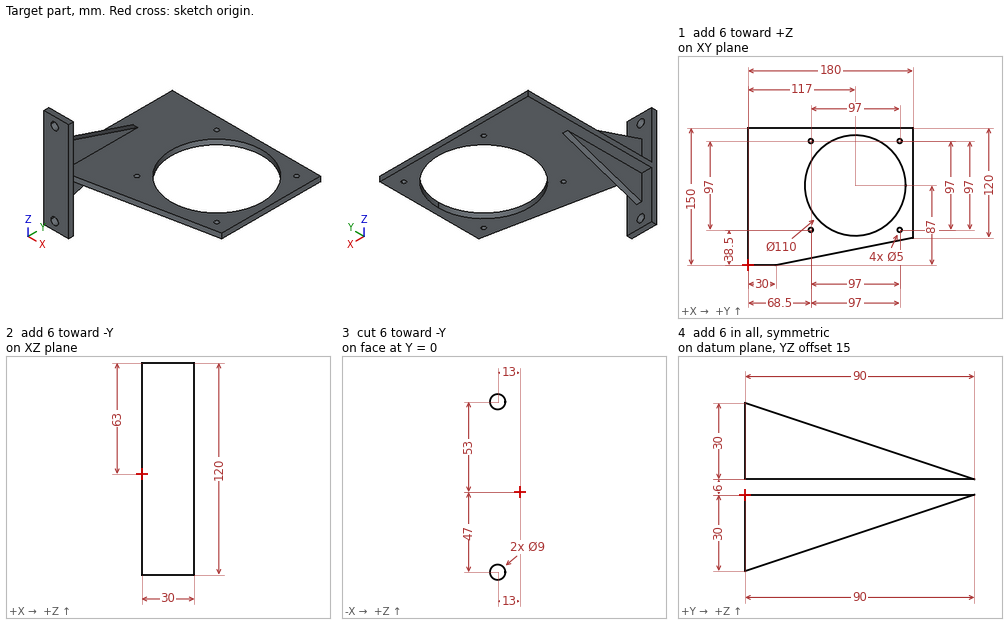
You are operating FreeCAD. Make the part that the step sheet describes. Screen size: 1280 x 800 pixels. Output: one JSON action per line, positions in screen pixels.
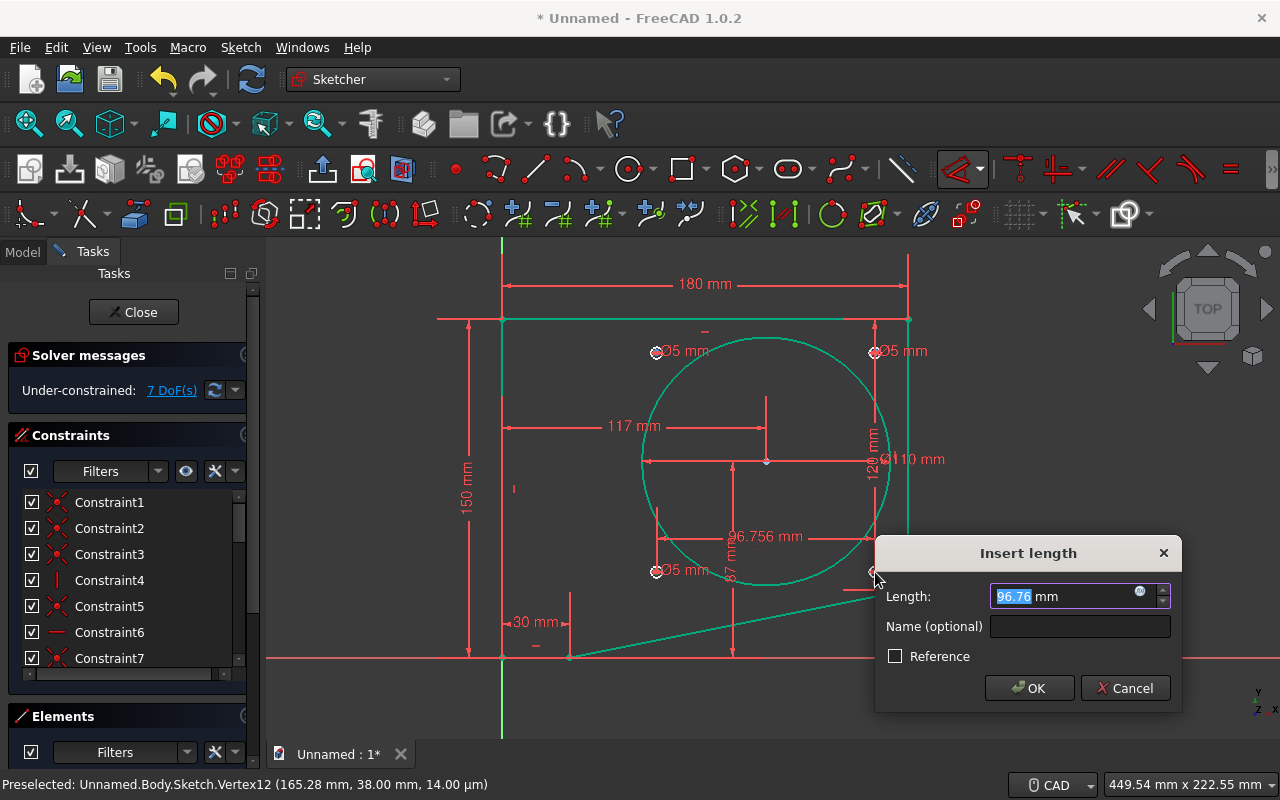
{"action": "type", "text": "97"}
{"action": "key", "text": "Return"}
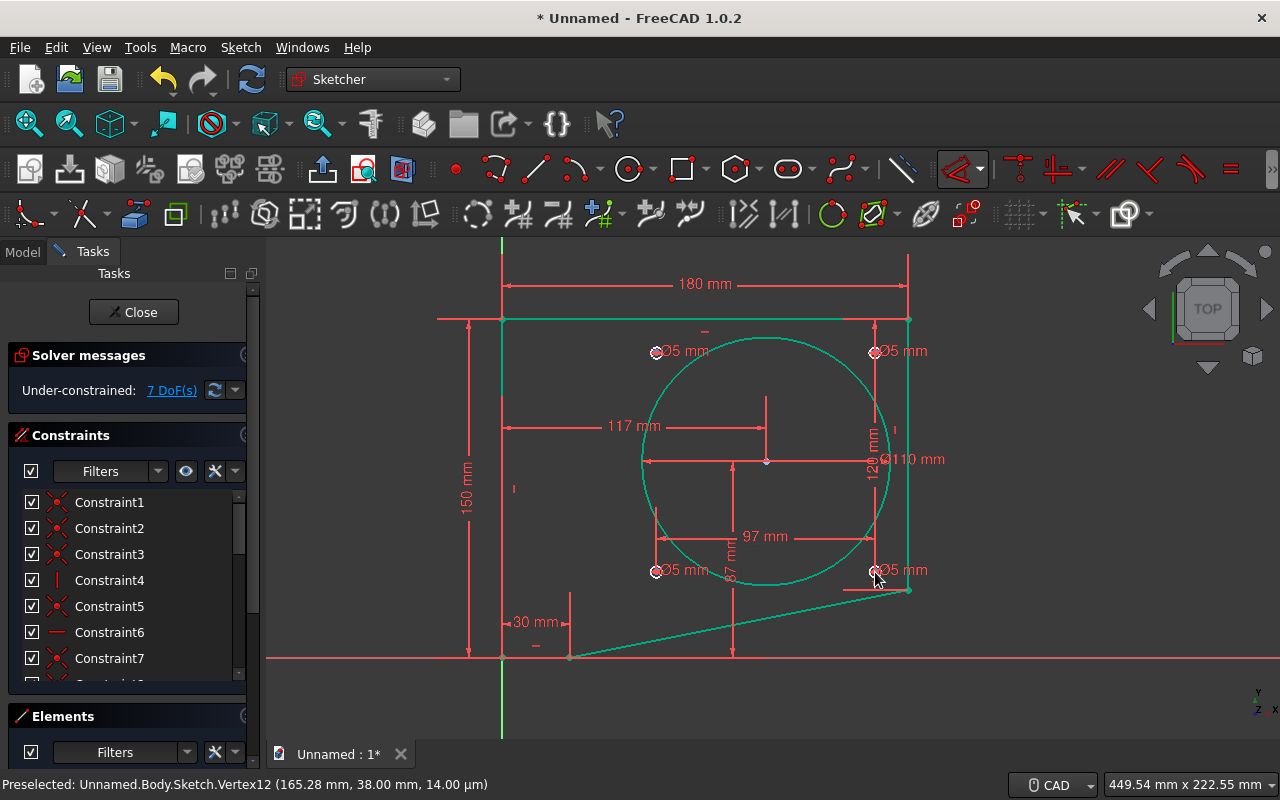
{"action": "left_click", "coordinate": [875, 572]}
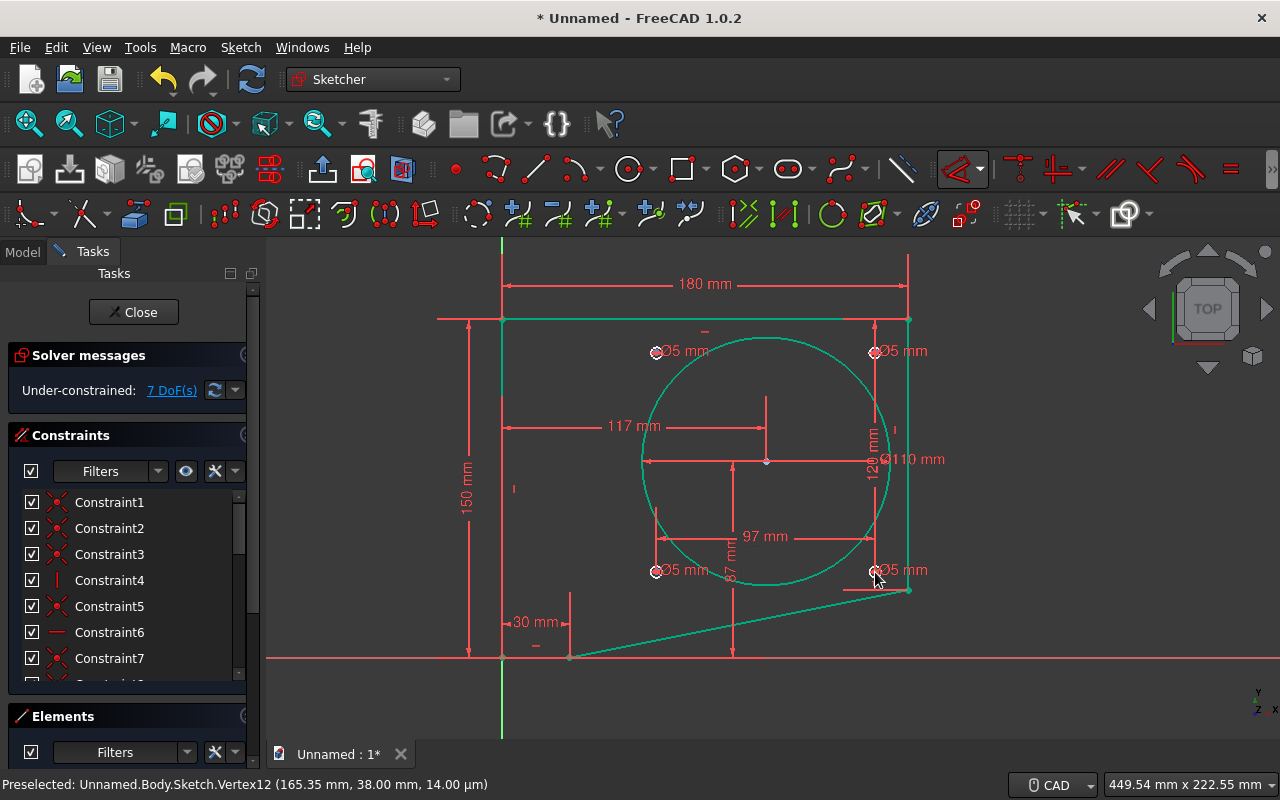
{"action": "left_click", "coordinate": [657, 353]}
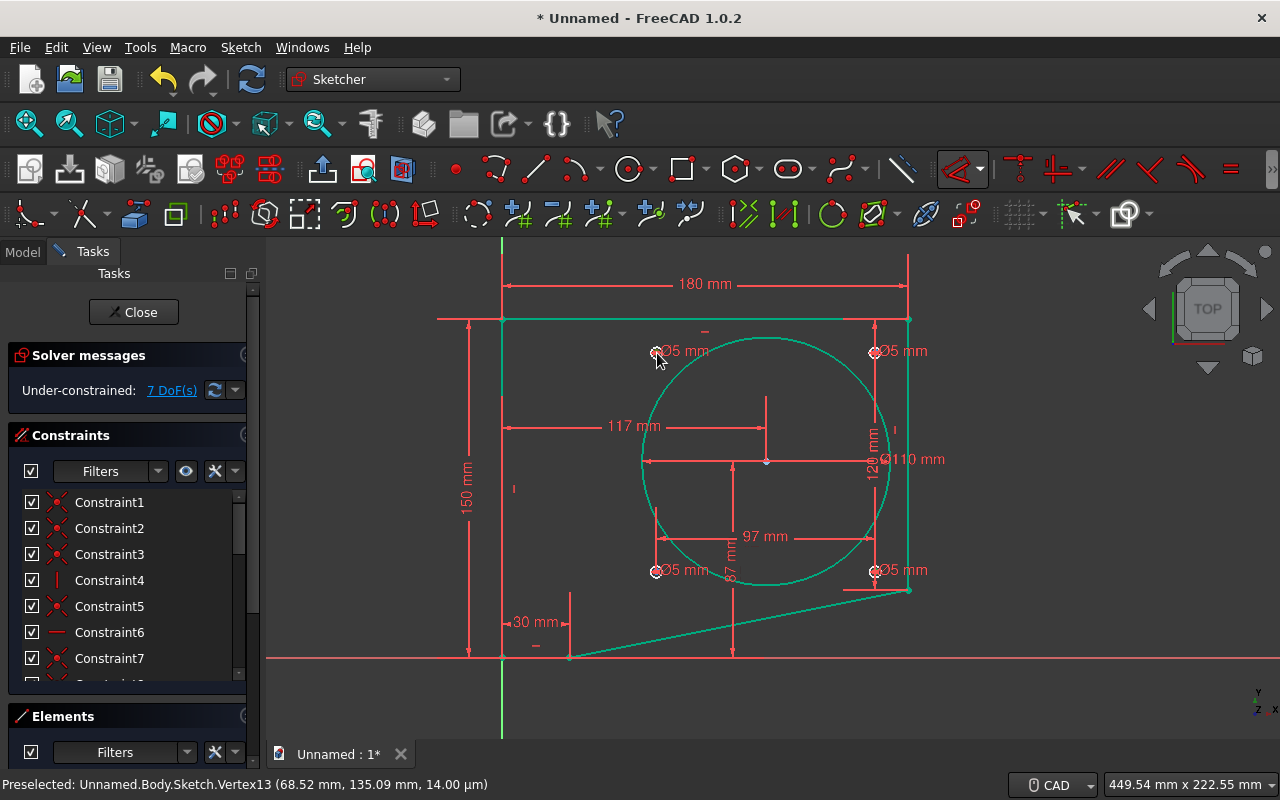
{"action": "key", "text": "l"}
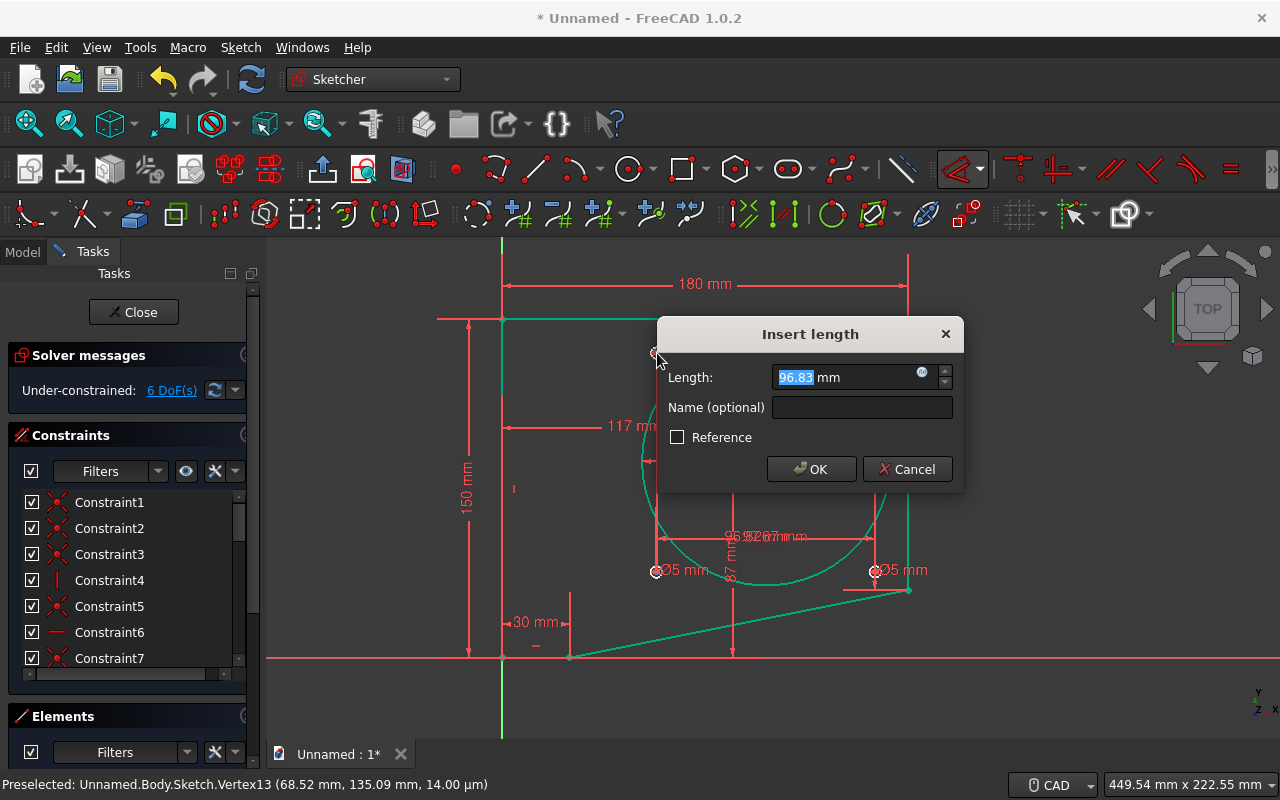
{"action": "type", "text": "97"}
{"action": "key", "text": "Return"}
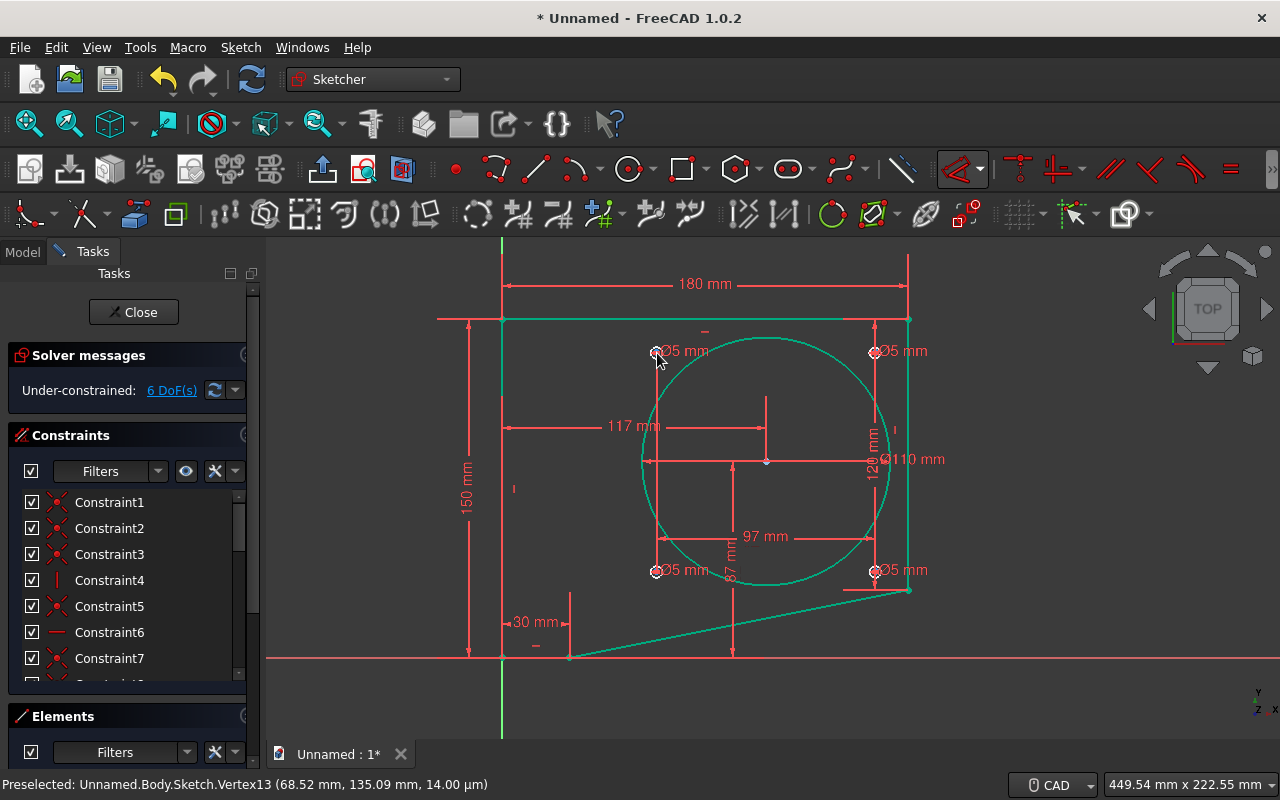
{"action": "left_click", "coordinate": [657, 572]}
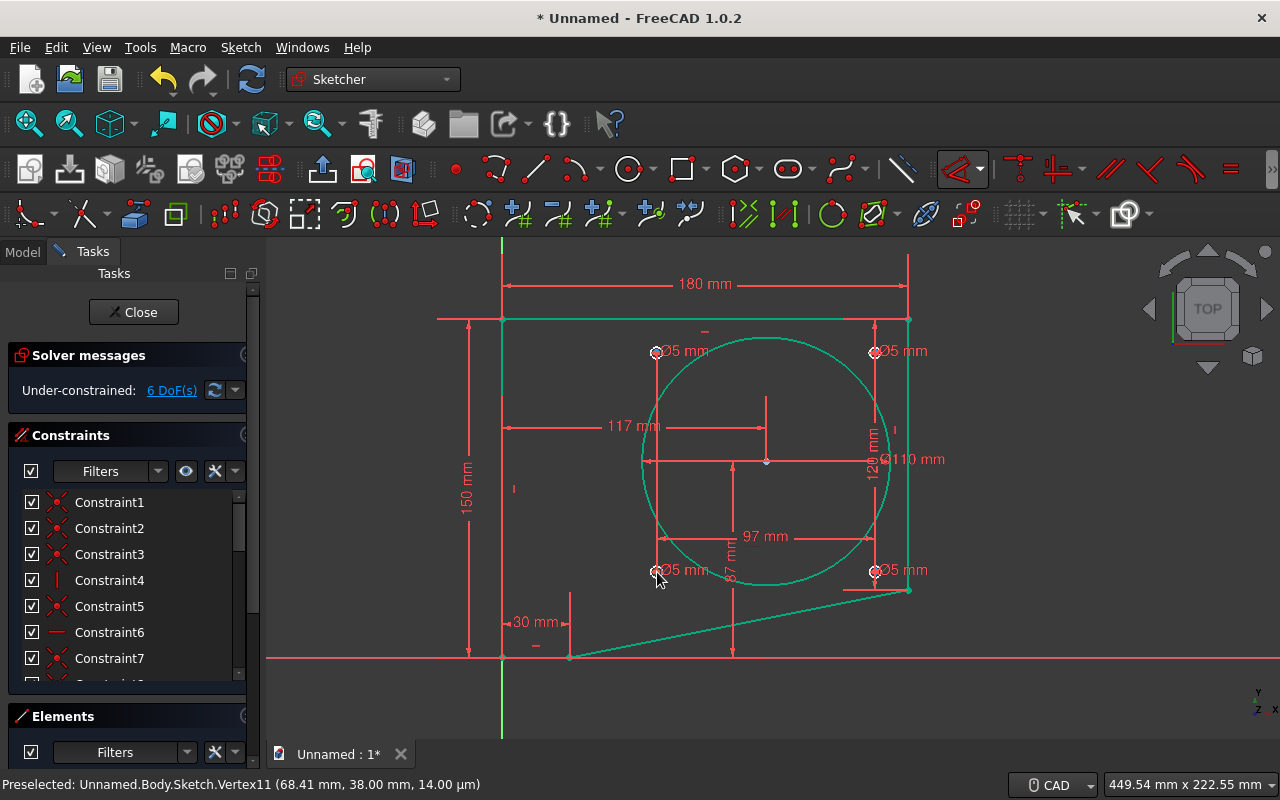
{"action": "left_click", "coordinate": [657, 353]}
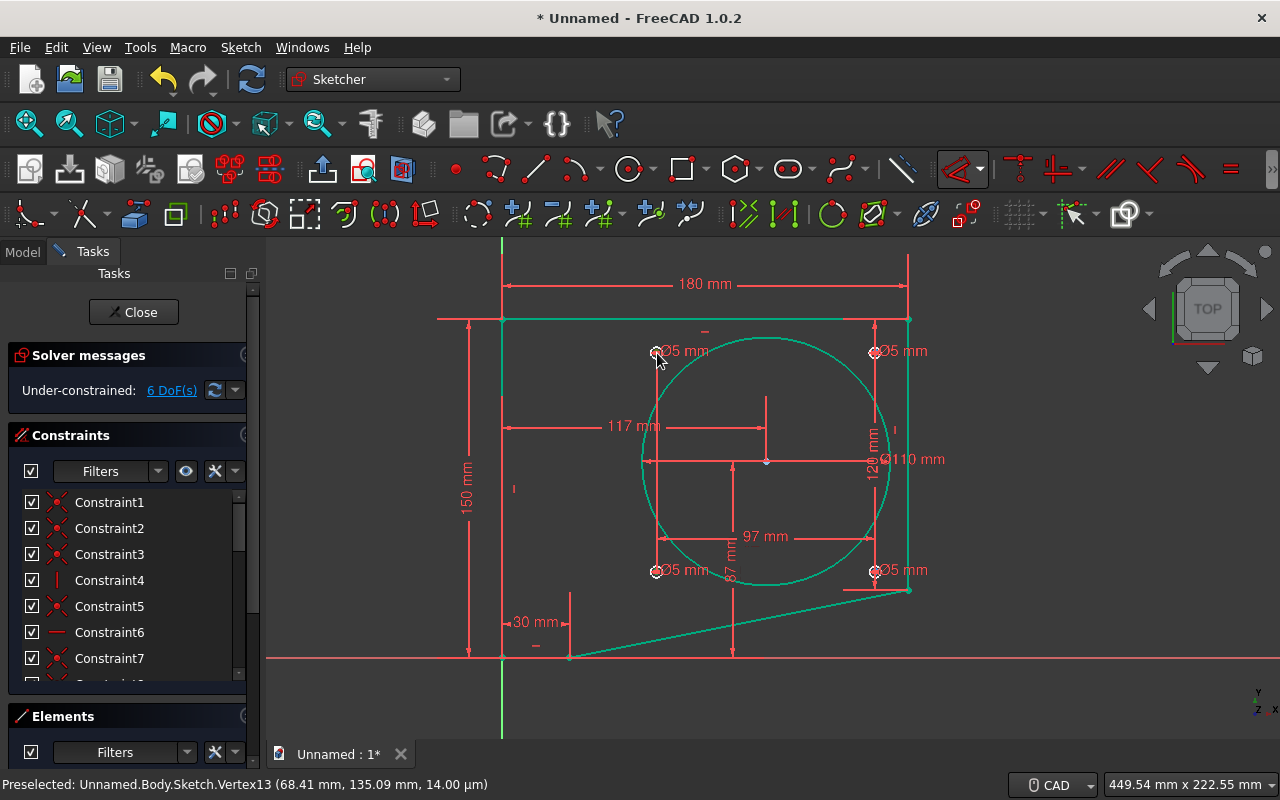
{"action": "key", "text": "i"}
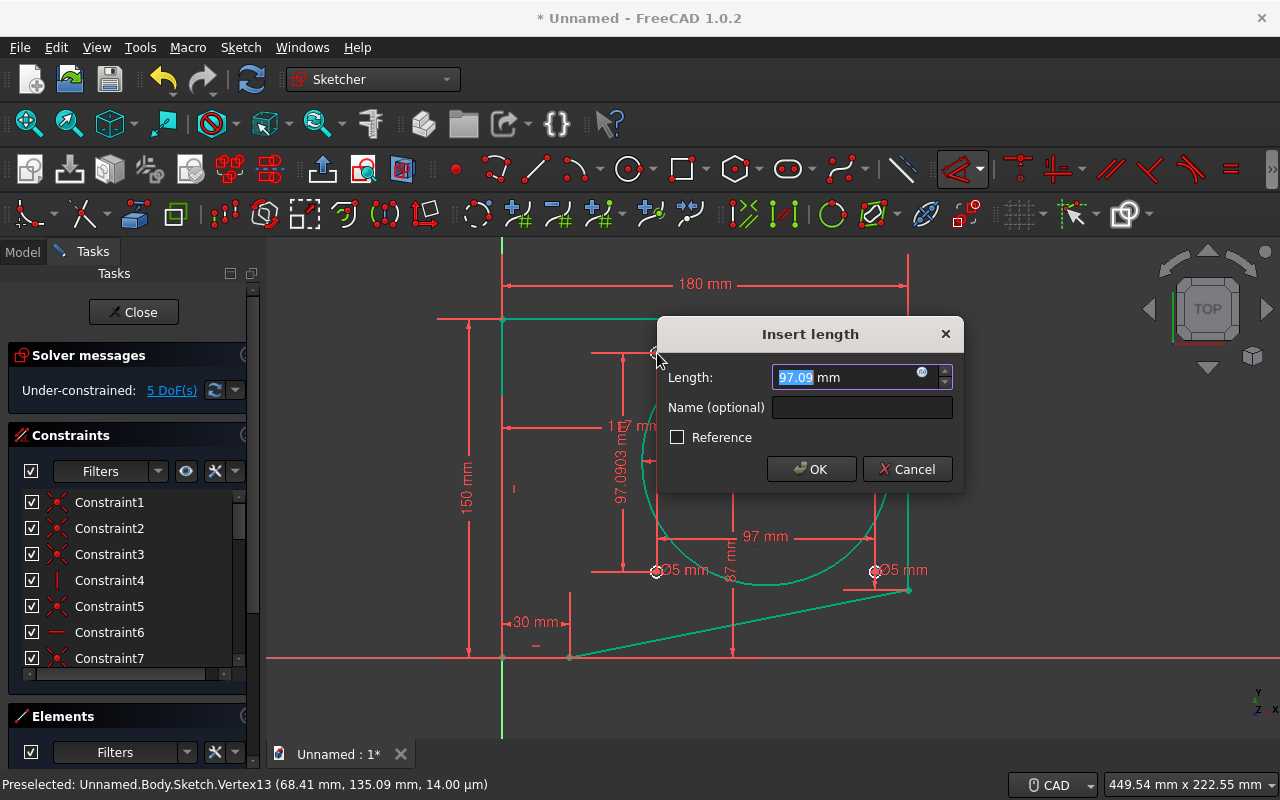
{"action": "type", "text": "97"}
{"action": "key", "text": "Return"}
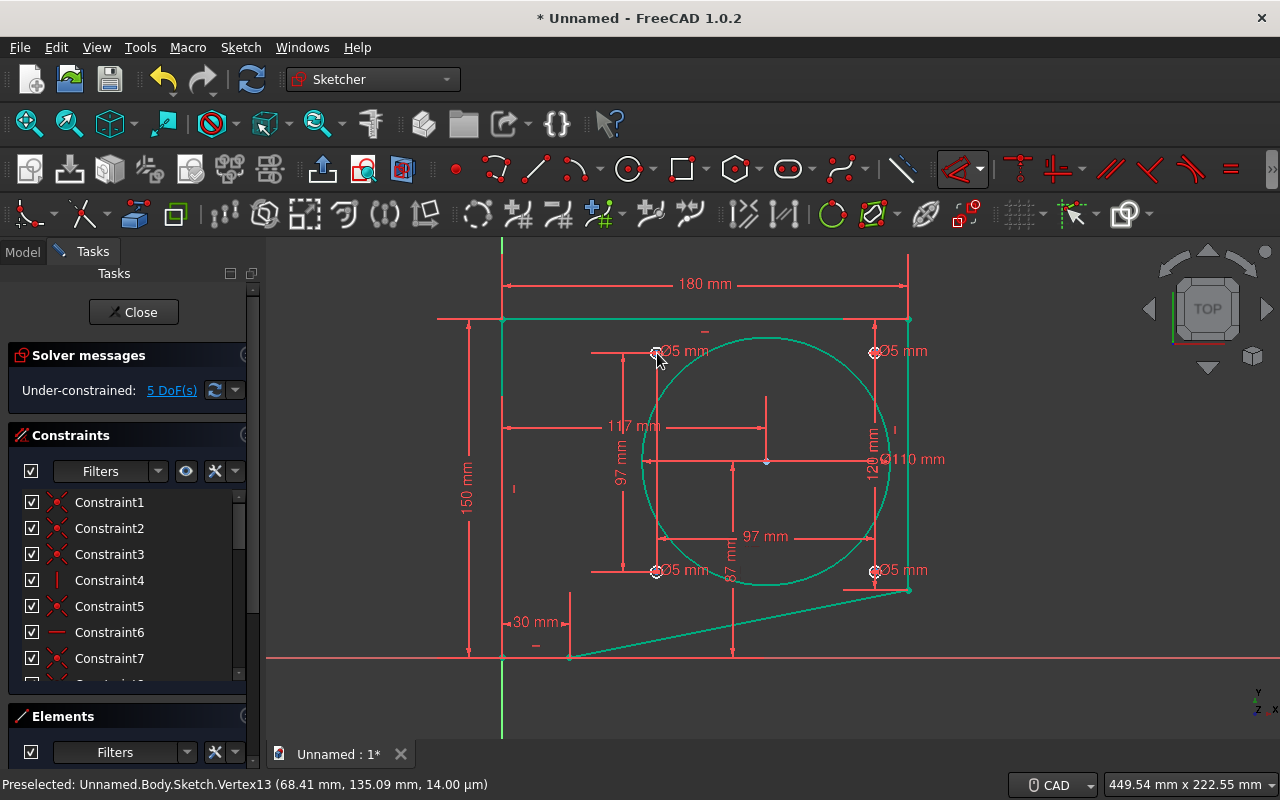
{"action": "left_click", "coordinate": [875, 572]}